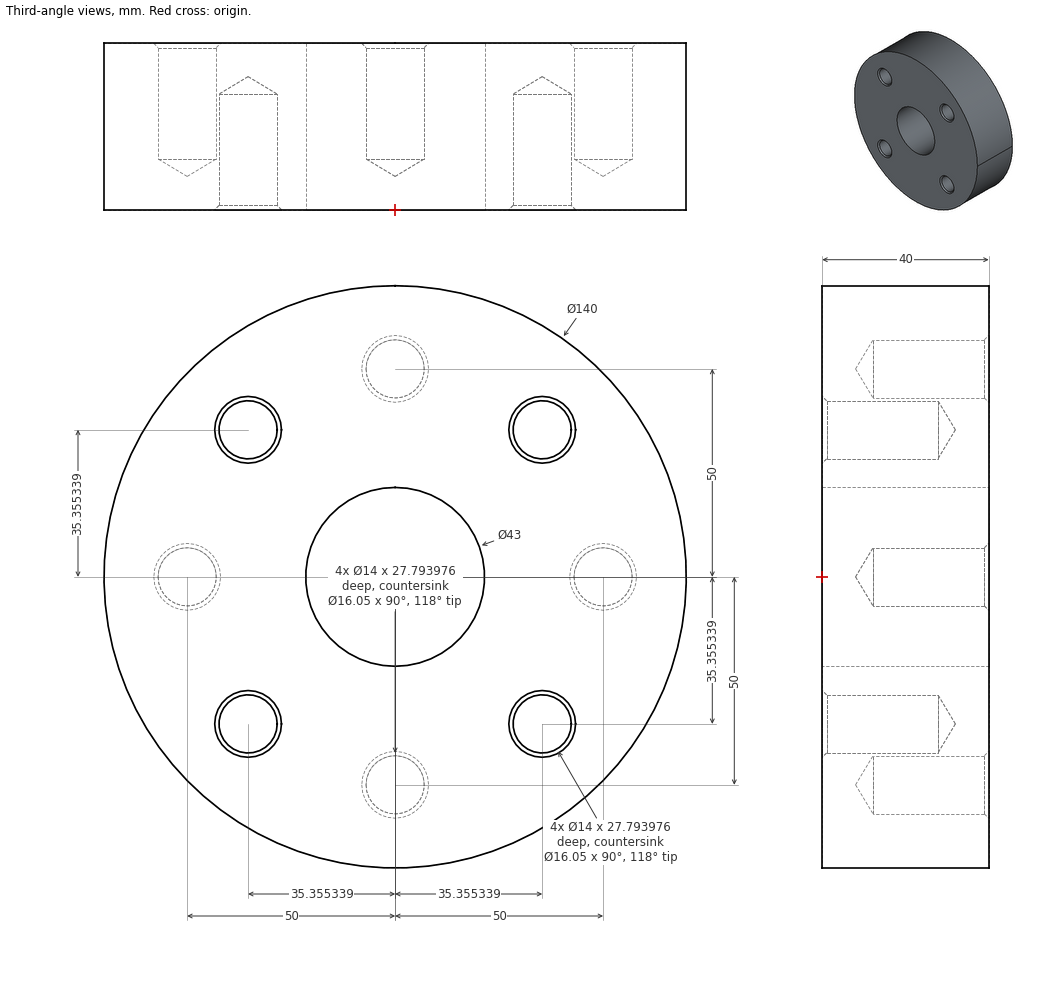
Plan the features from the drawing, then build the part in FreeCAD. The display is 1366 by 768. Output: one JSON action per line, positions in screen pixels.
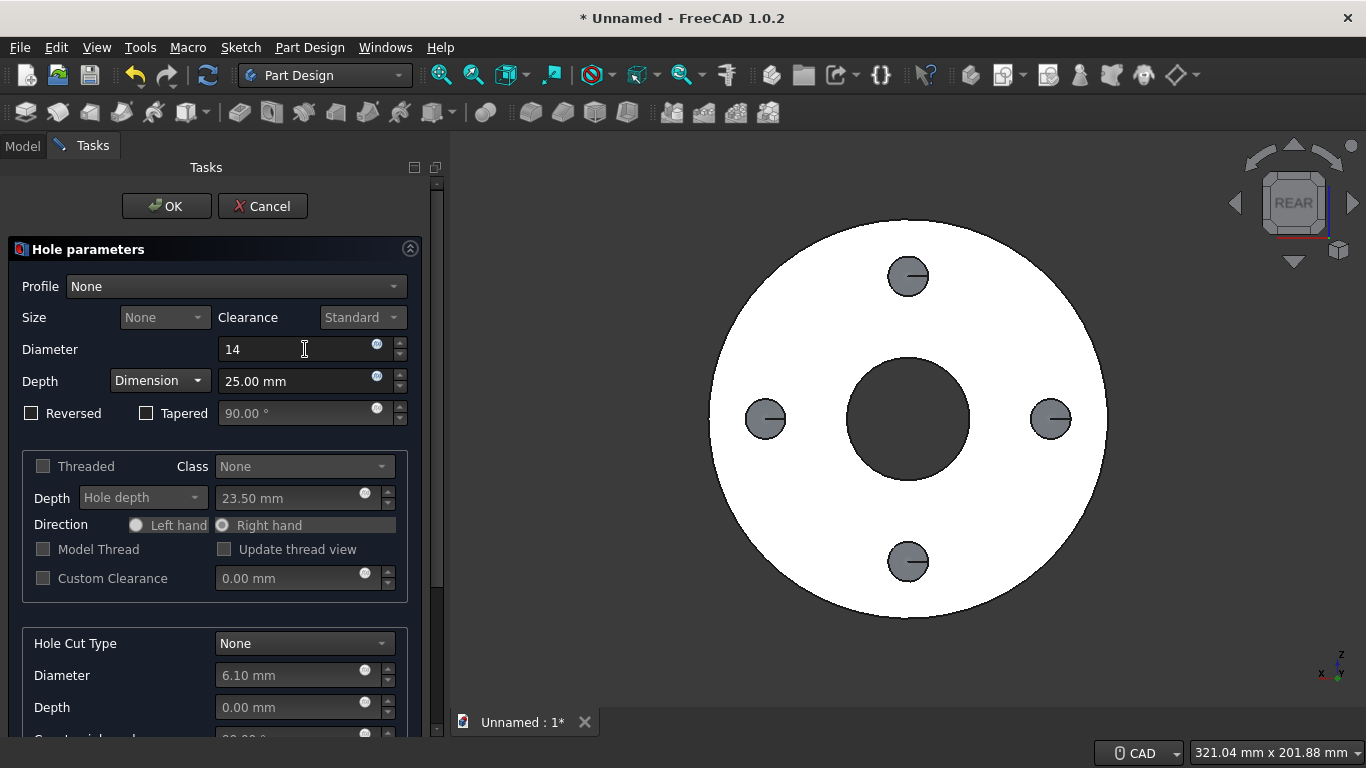
{"action": "triple_click", "coordinate": [305, 381]}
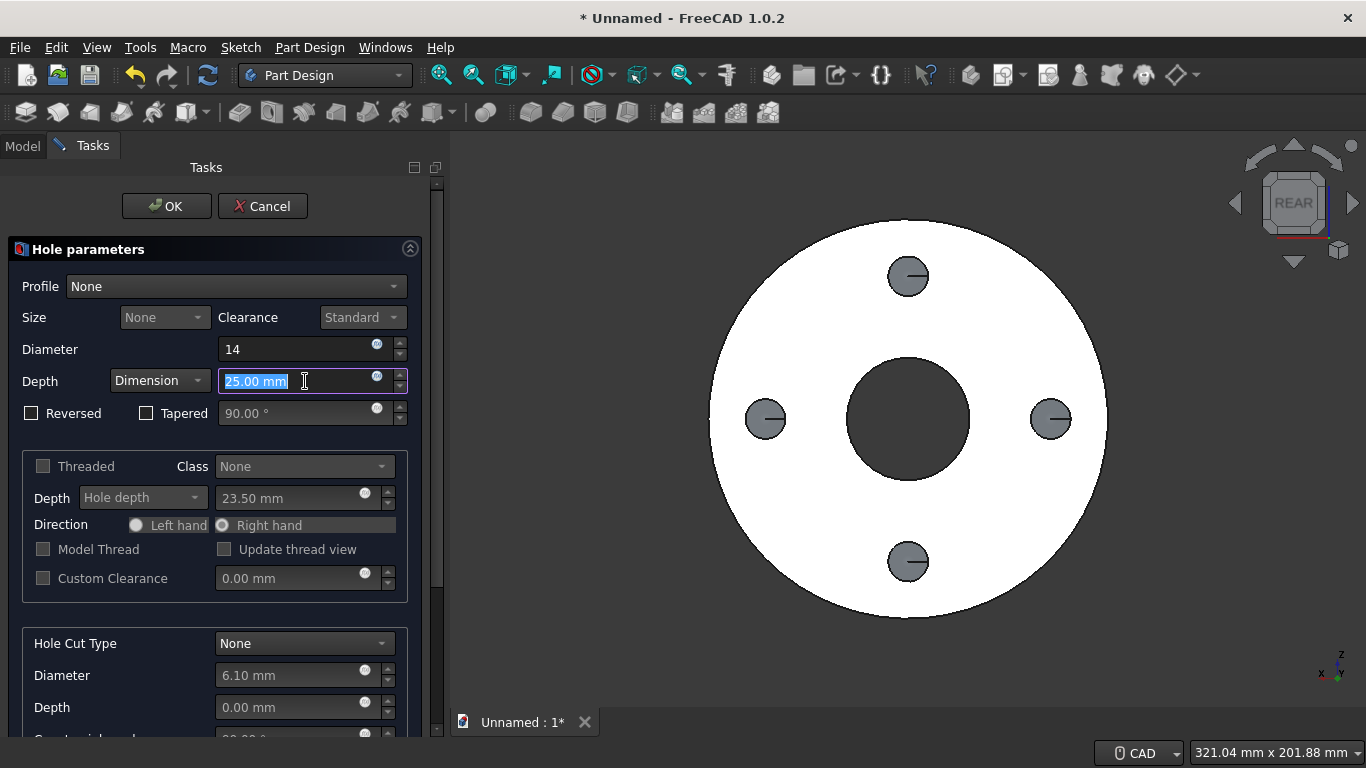
{"action": "type", "text": "27.793976"}
{"action": "key", "text": "Tab"}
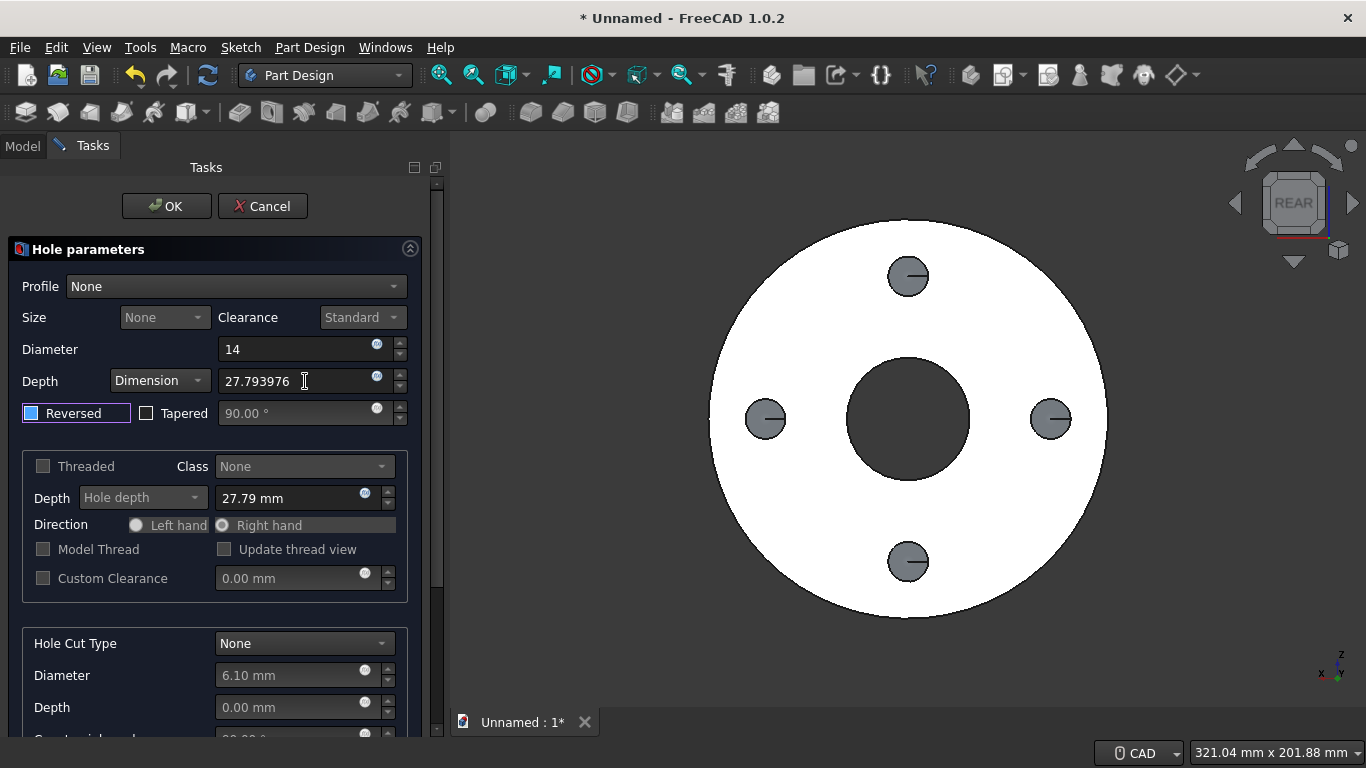
{"action": "left_click", "coordinate": [306, 644]}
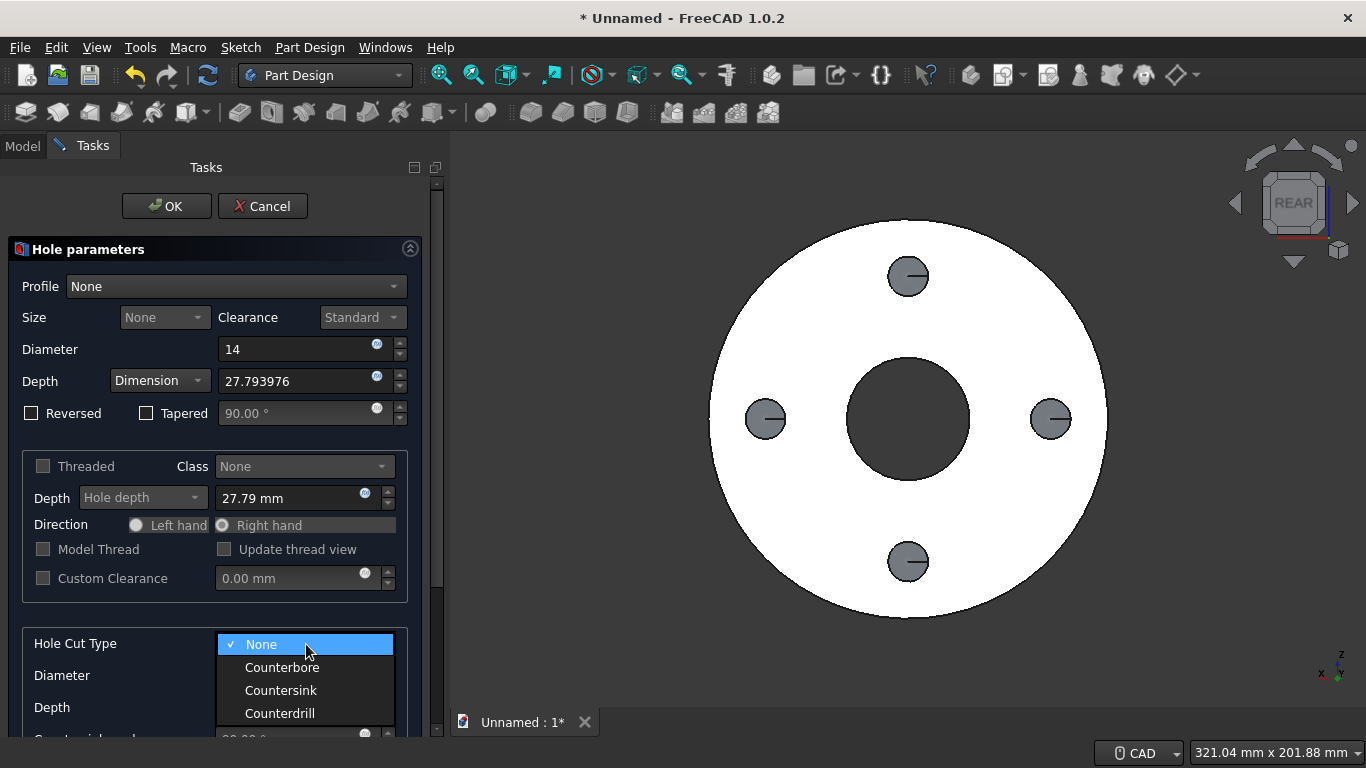
{"action": "left_click", "coordinate": [304, 690]}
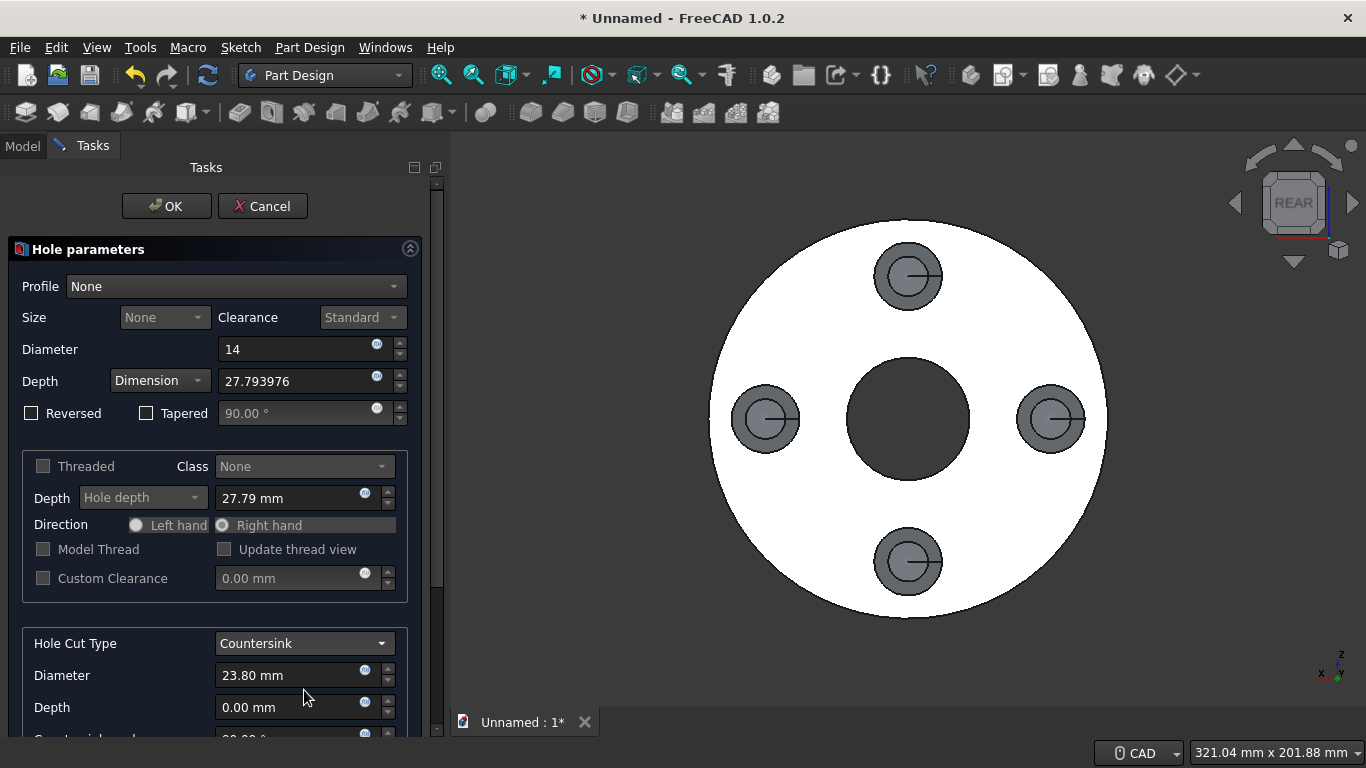
{"action": "triple_click", "coordinate": [298, 675]}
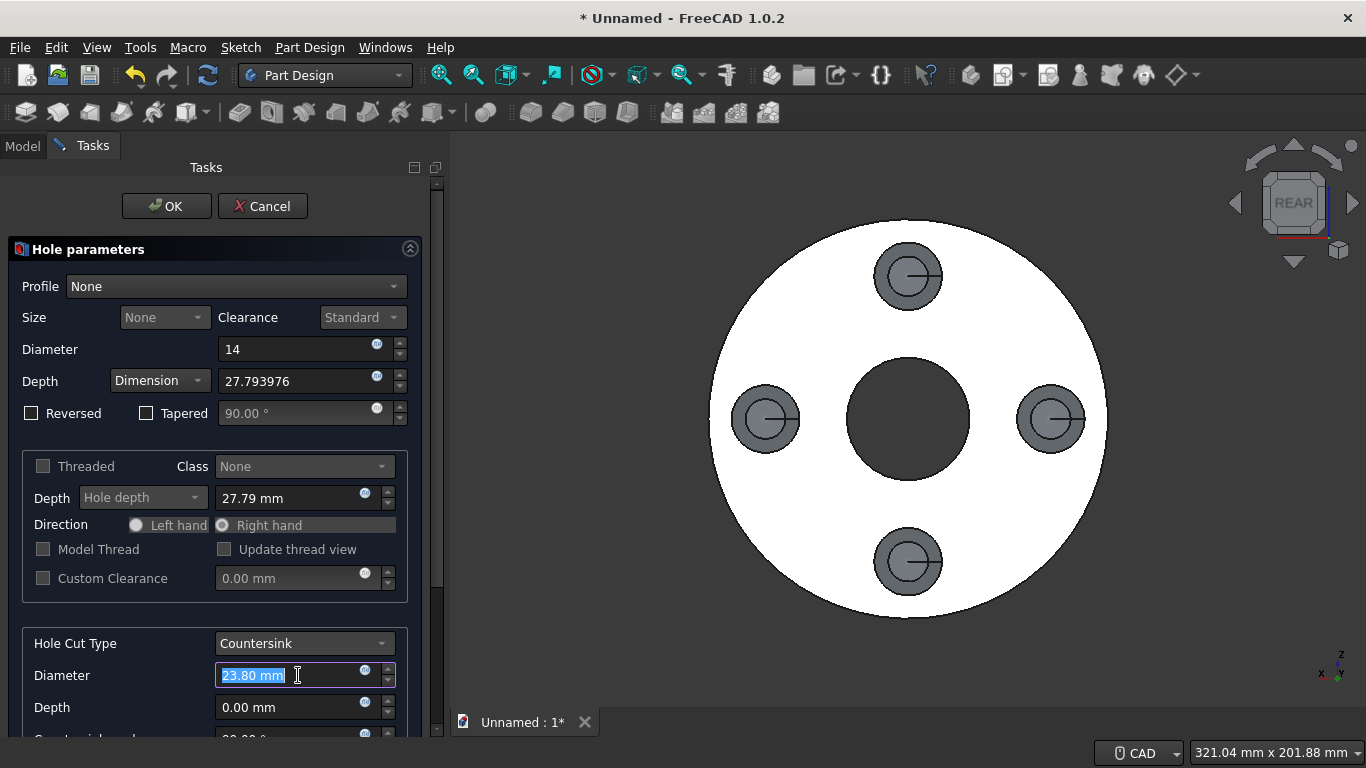
{"action": "type", "text": "16.05"}
{"action": "key", "text": "Tab"}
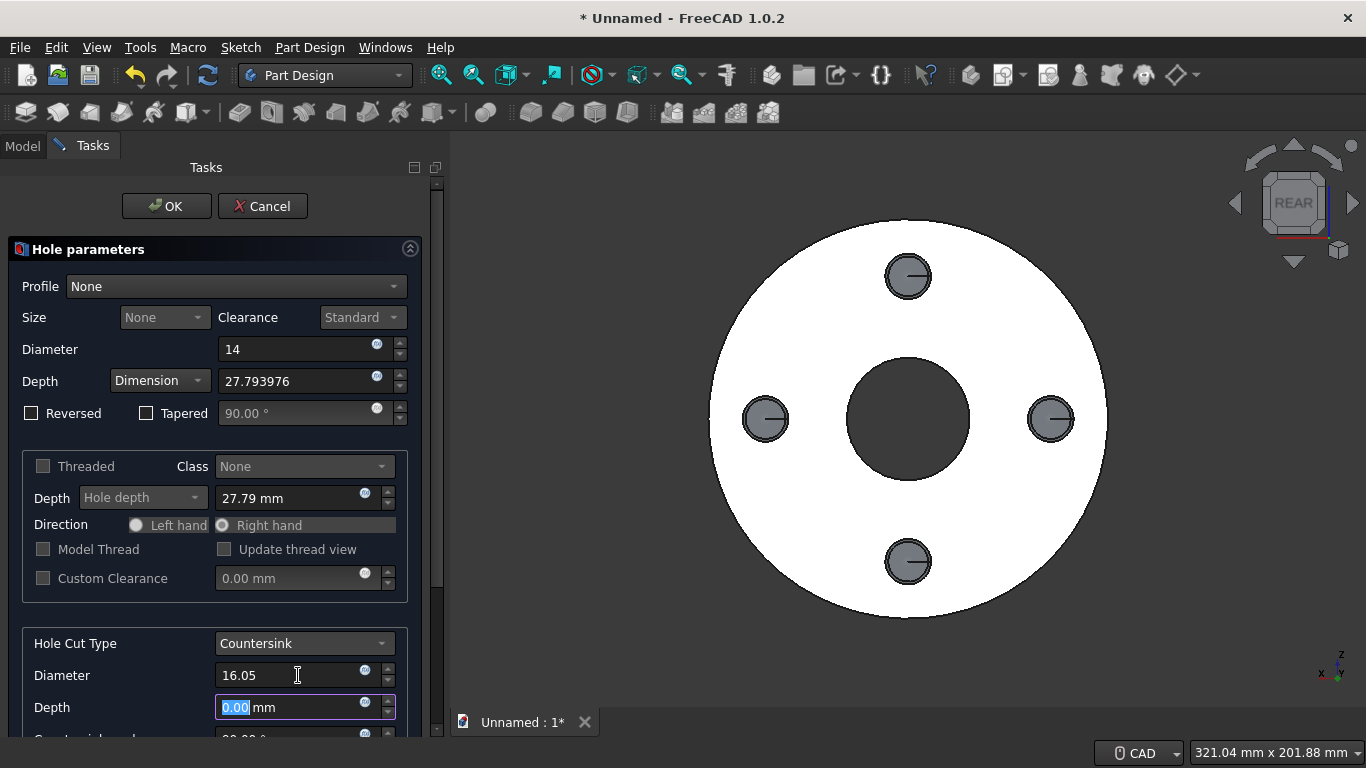
{"action": "left_click", "coordinate": [167, 206]}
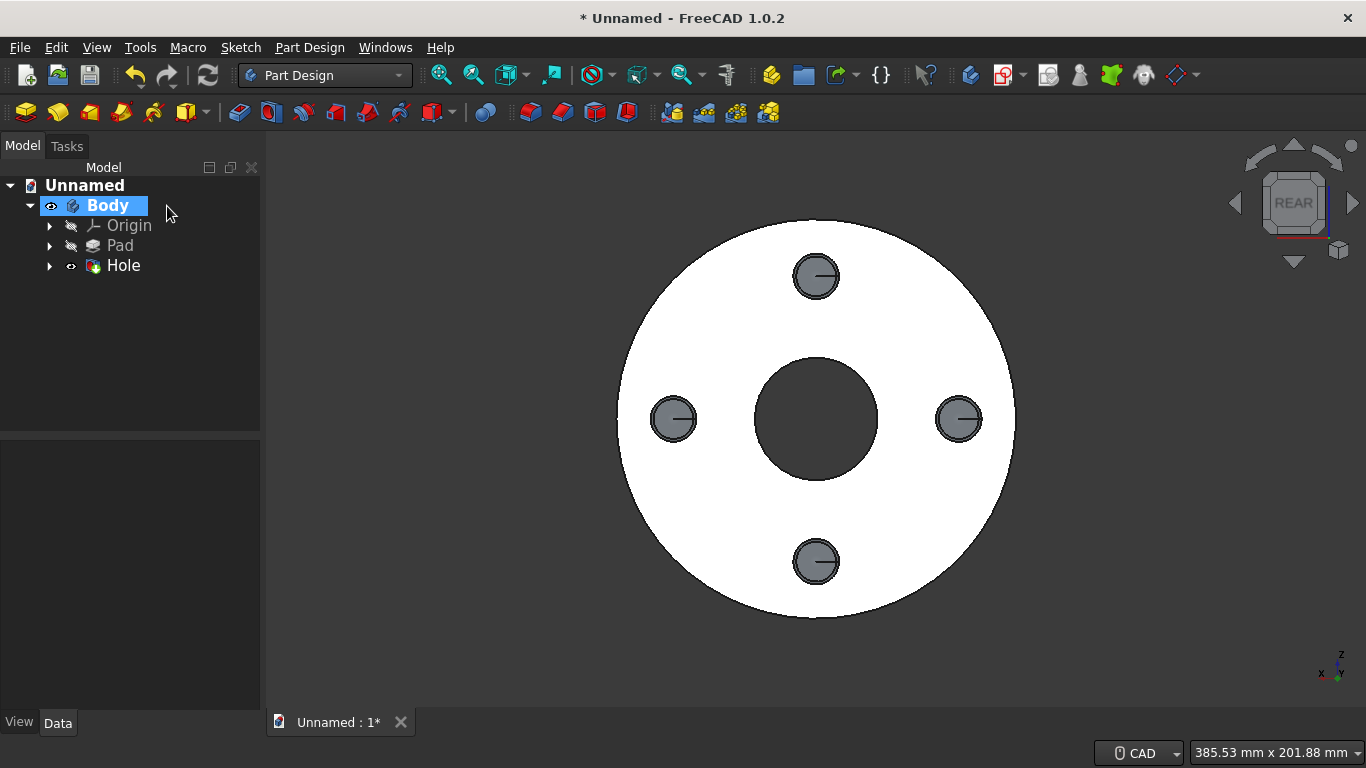
{"action": "left_click", "coordinate": [1004, 76]}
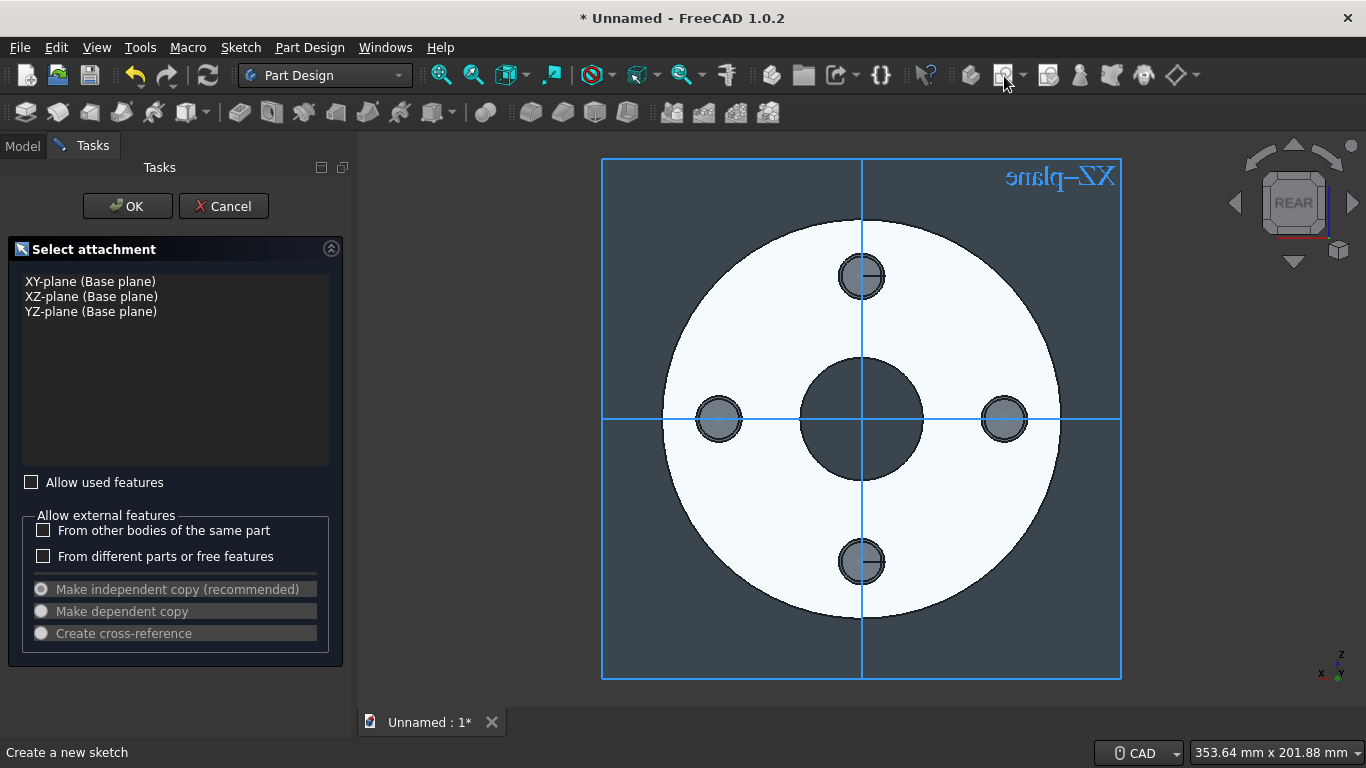
{"action": "left_click", "coordinate": [82, 296]}